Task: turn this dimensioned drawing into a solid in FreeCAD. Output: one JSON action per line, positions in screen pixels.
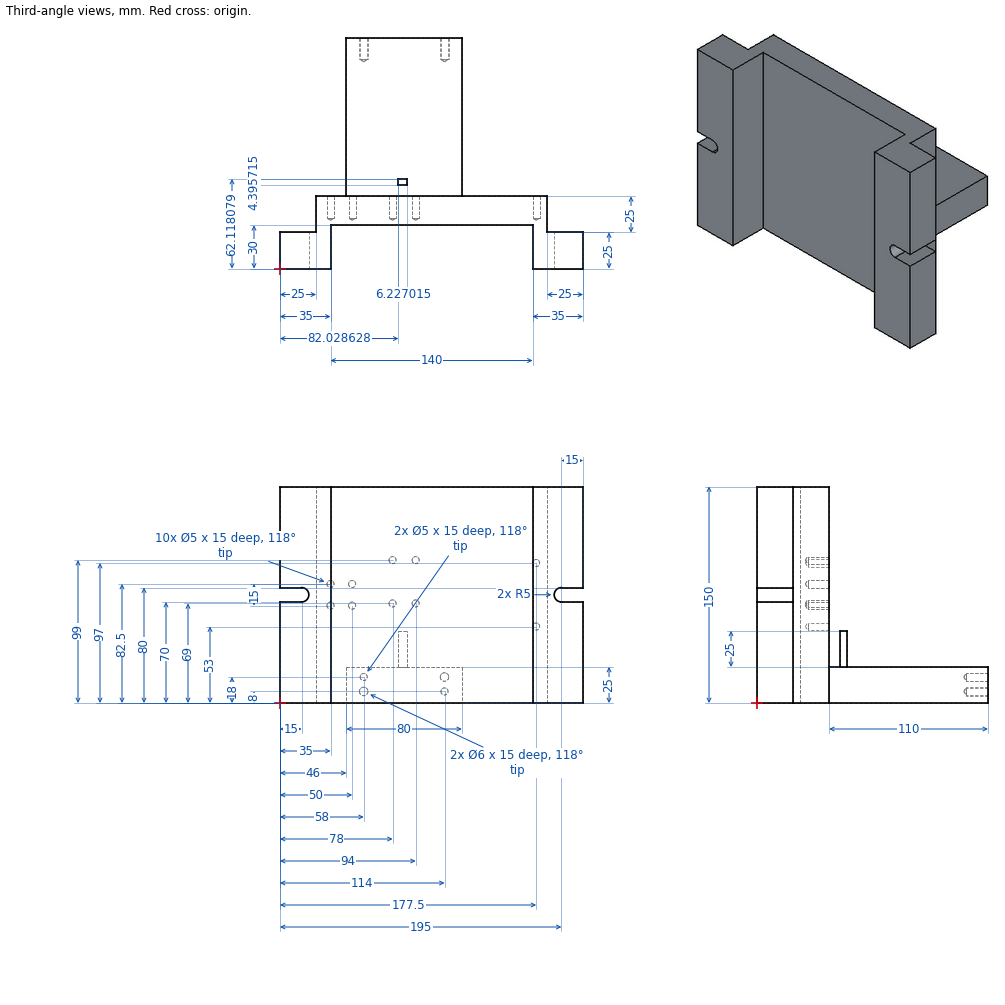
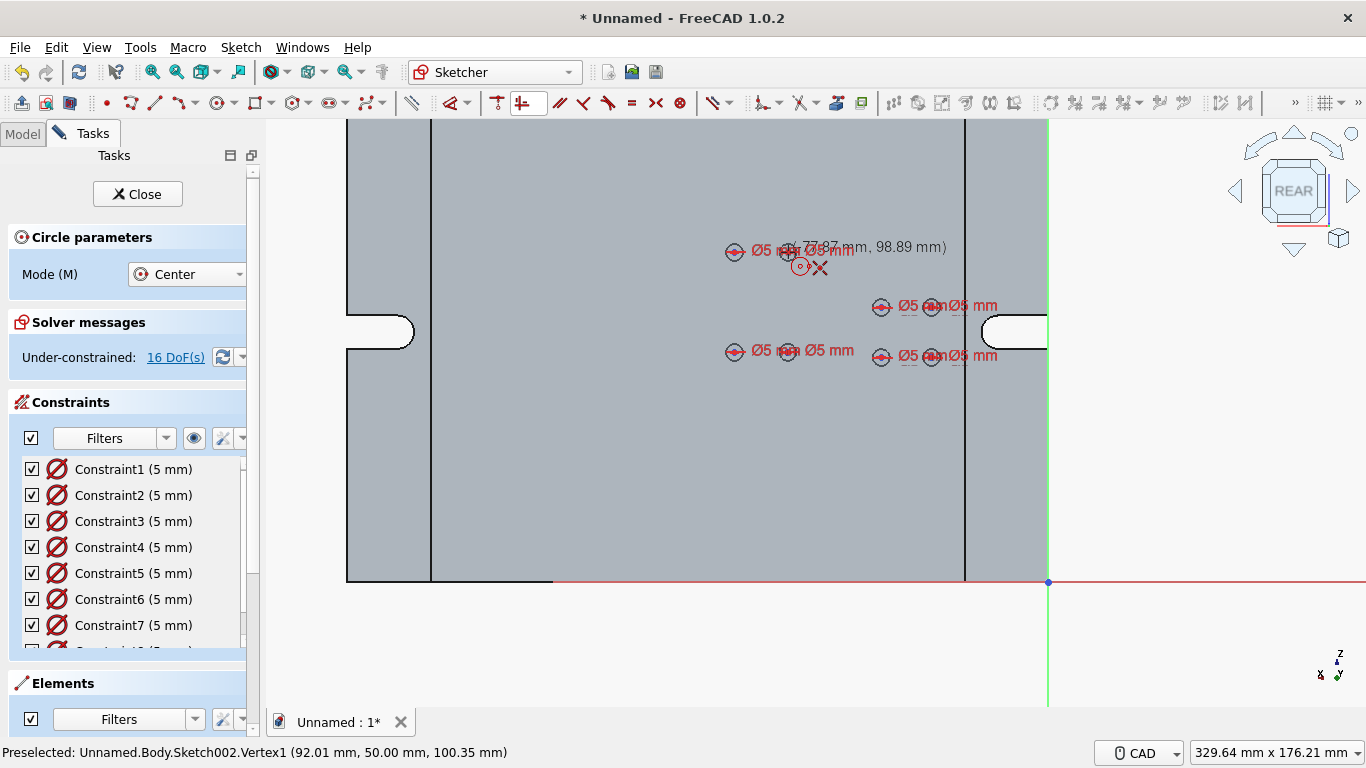
{"action": "scroll", "coordinate": [456, 259], "scroll_direction": "up", "scroll_amount": 6}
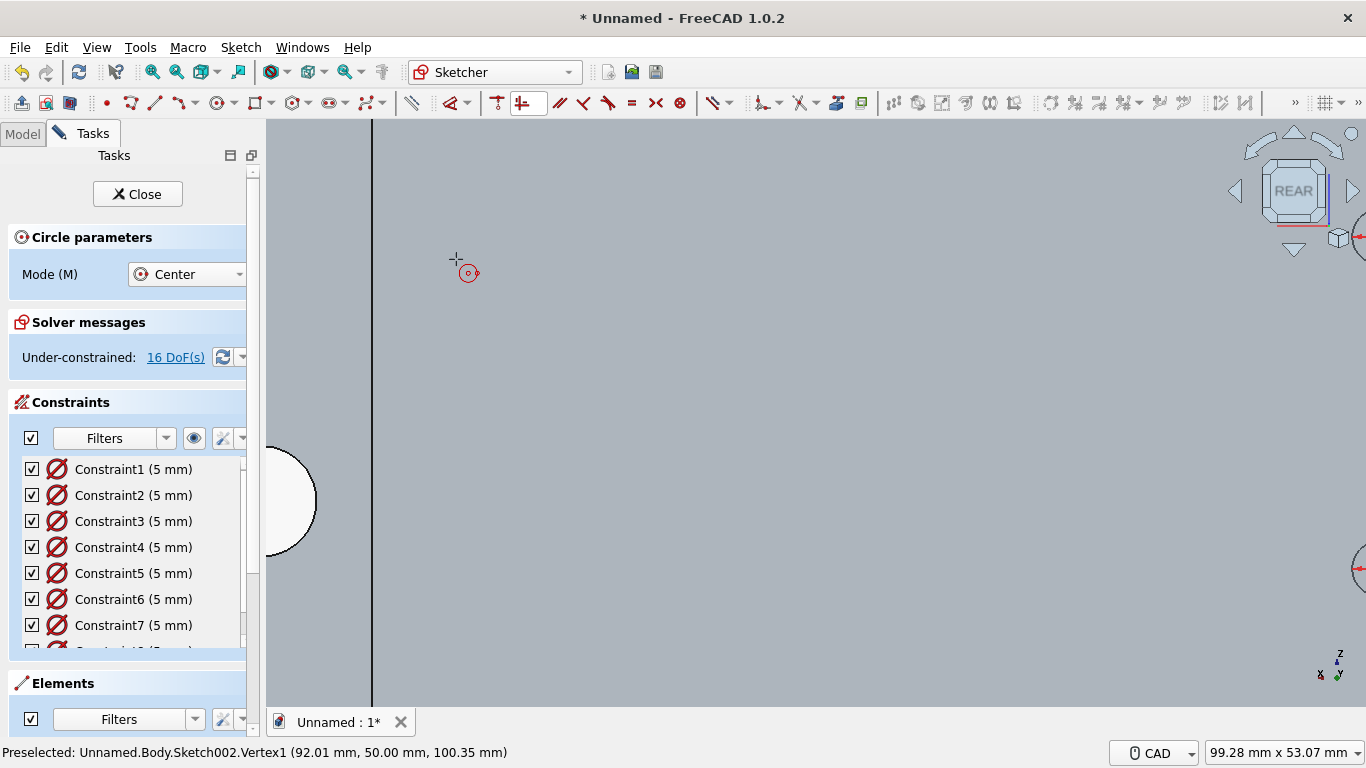
{"action": "left_click", "coordinate": [455, 258]}
{"action": "mouse_move", "coordinate": [475, 238]}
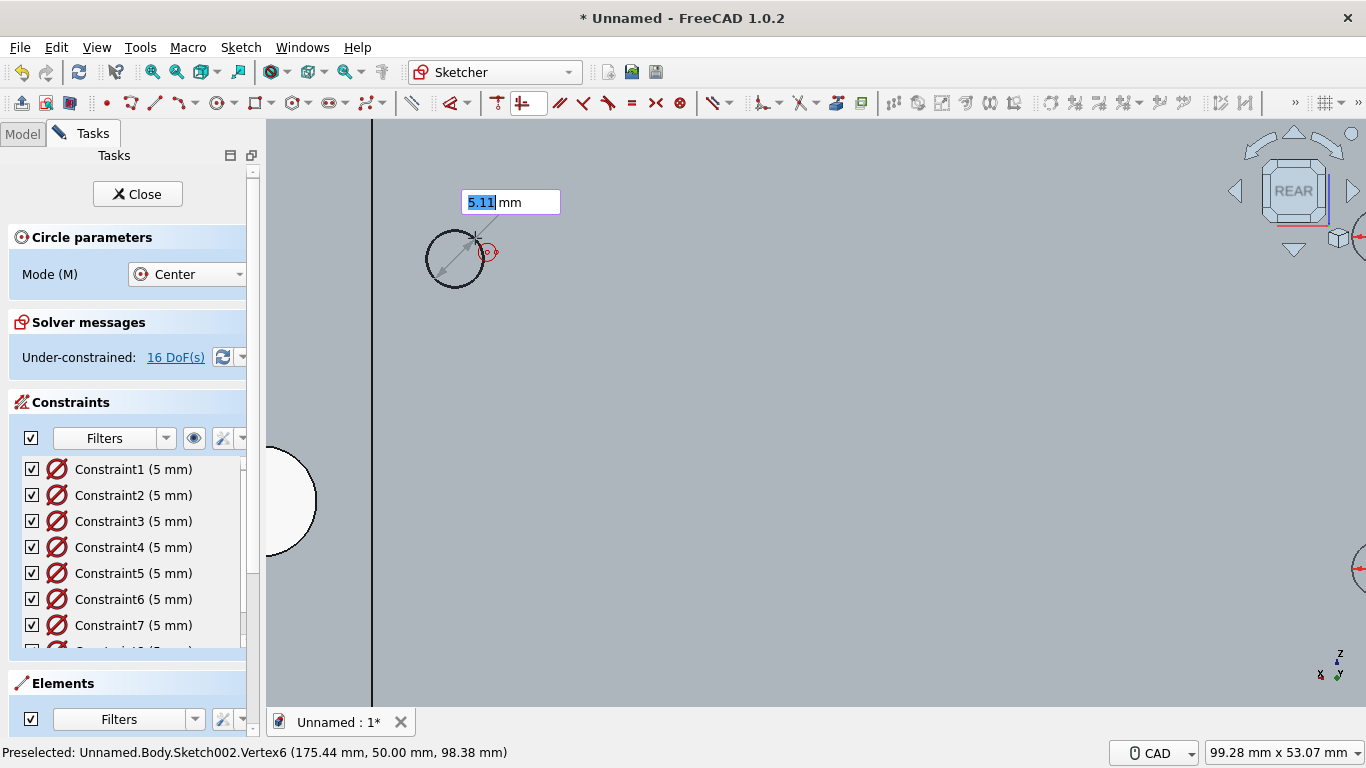
{"action": "type", "text": "5"}
{"action": "key", "text": "Return"}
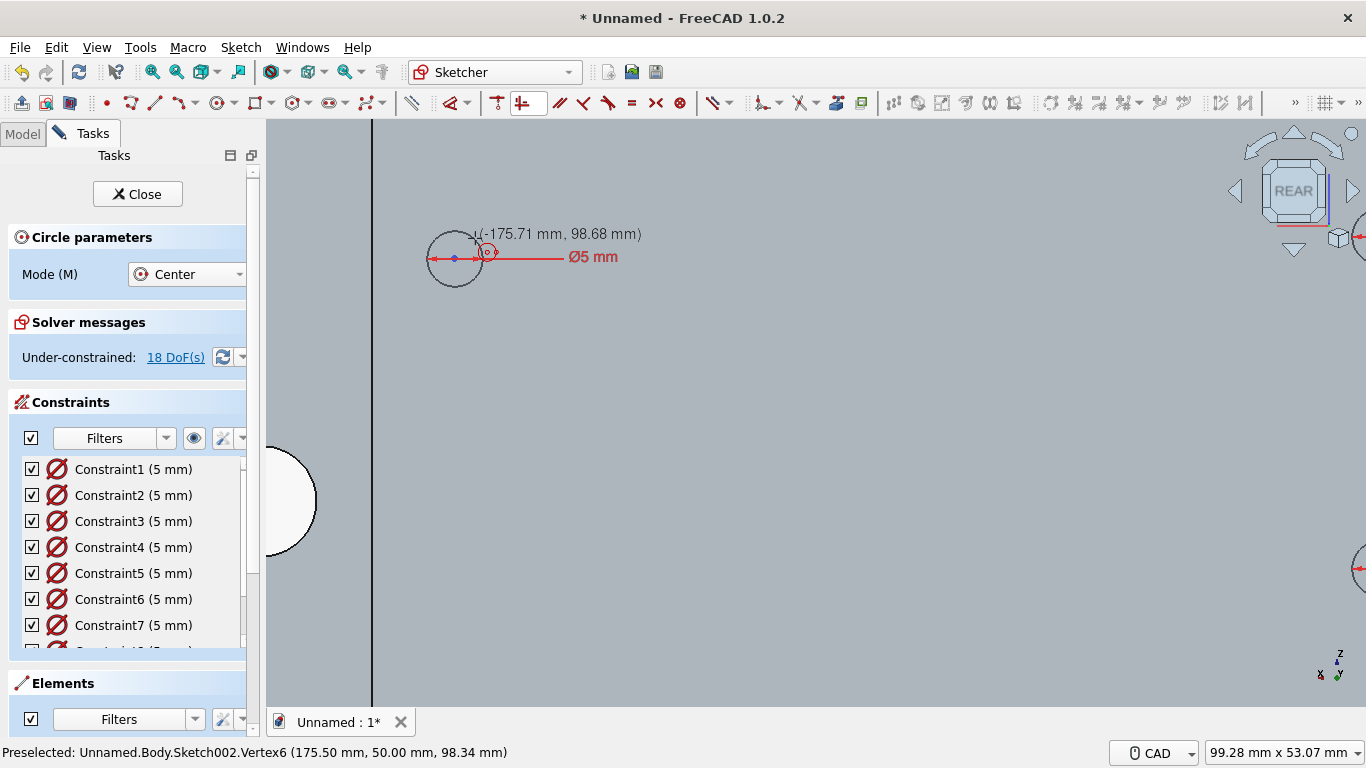
{"action": "scroll", "coordinate": [456, 259], "scroll_direction": "down", "scroll_amount": 6}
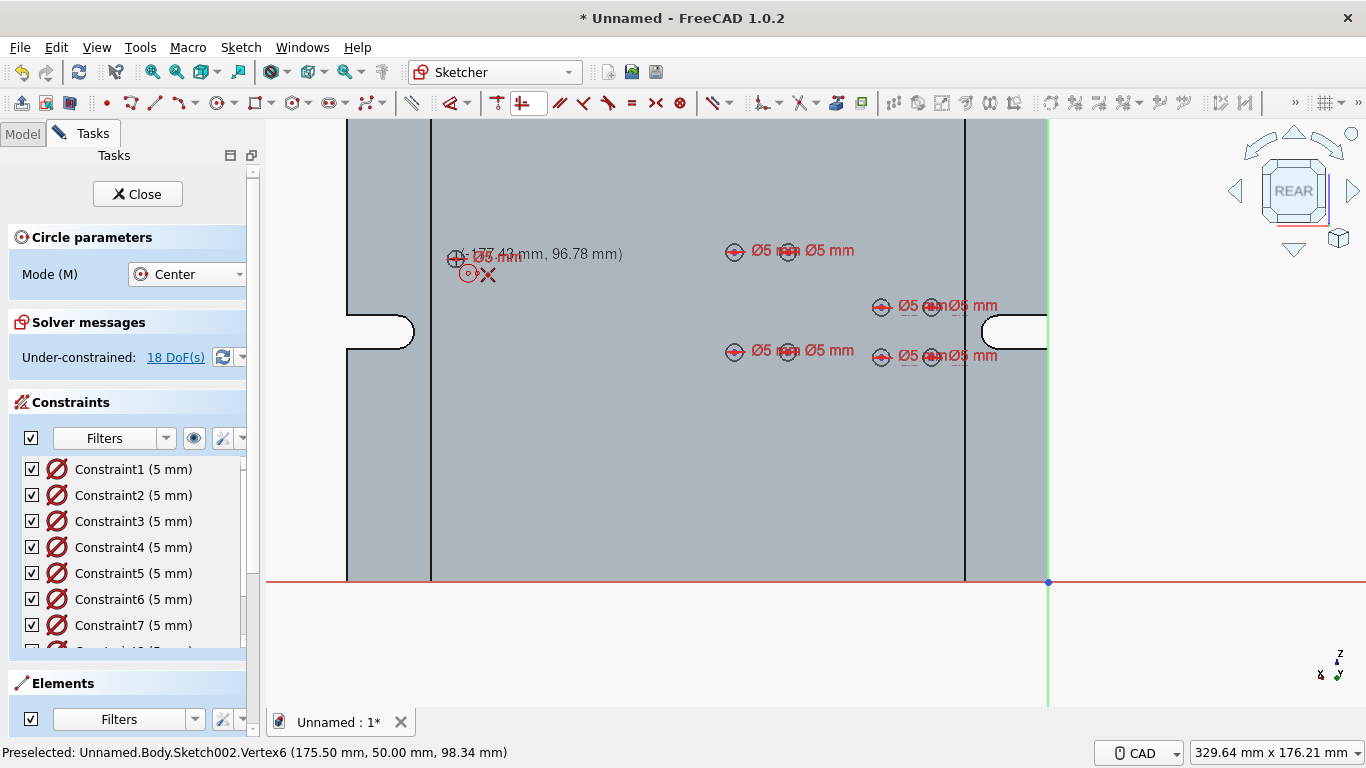
{"action": "scroll", "coordinate": [456, 406], "scroll_direction": "up", "scroll_amount": 6}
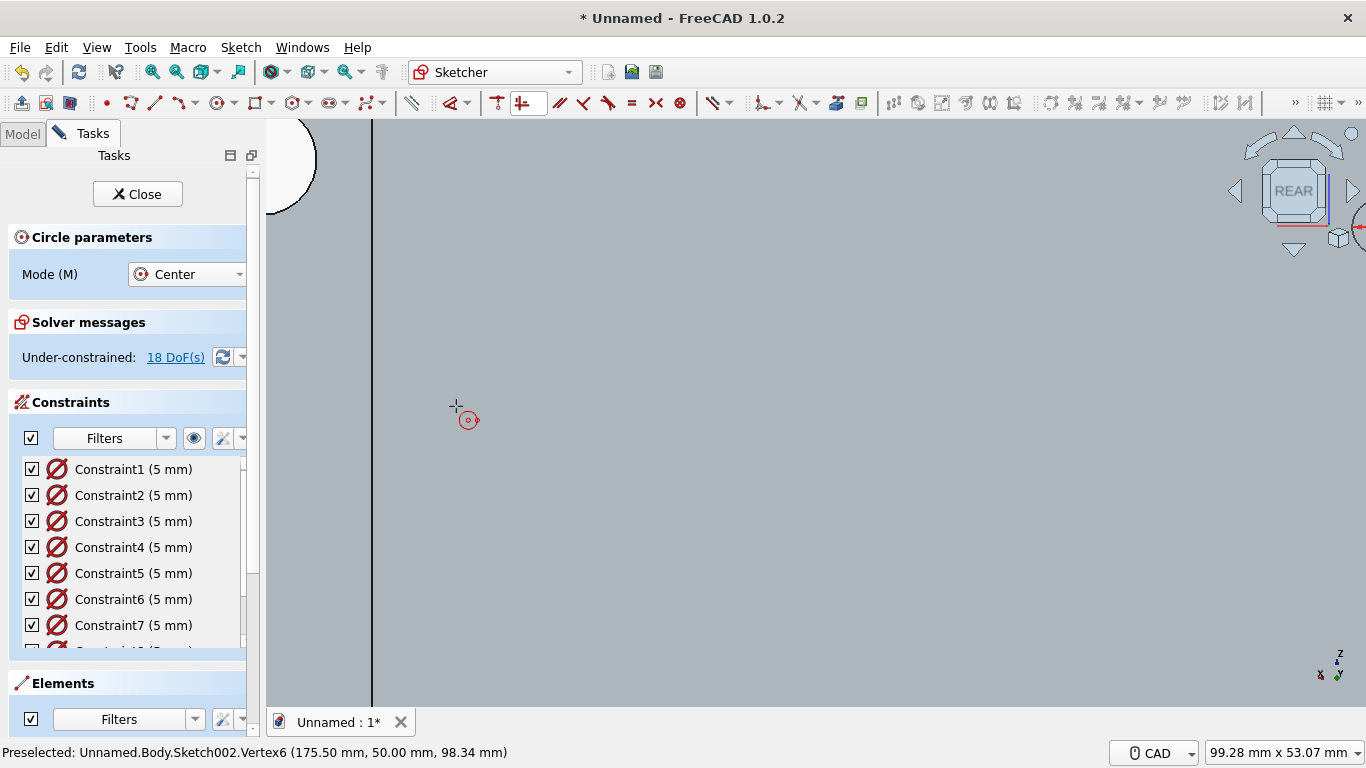
{"action": "left_click", "coordinate": [455, 403]}
{"action": "mouse_move", "coordinate": [475, 384]}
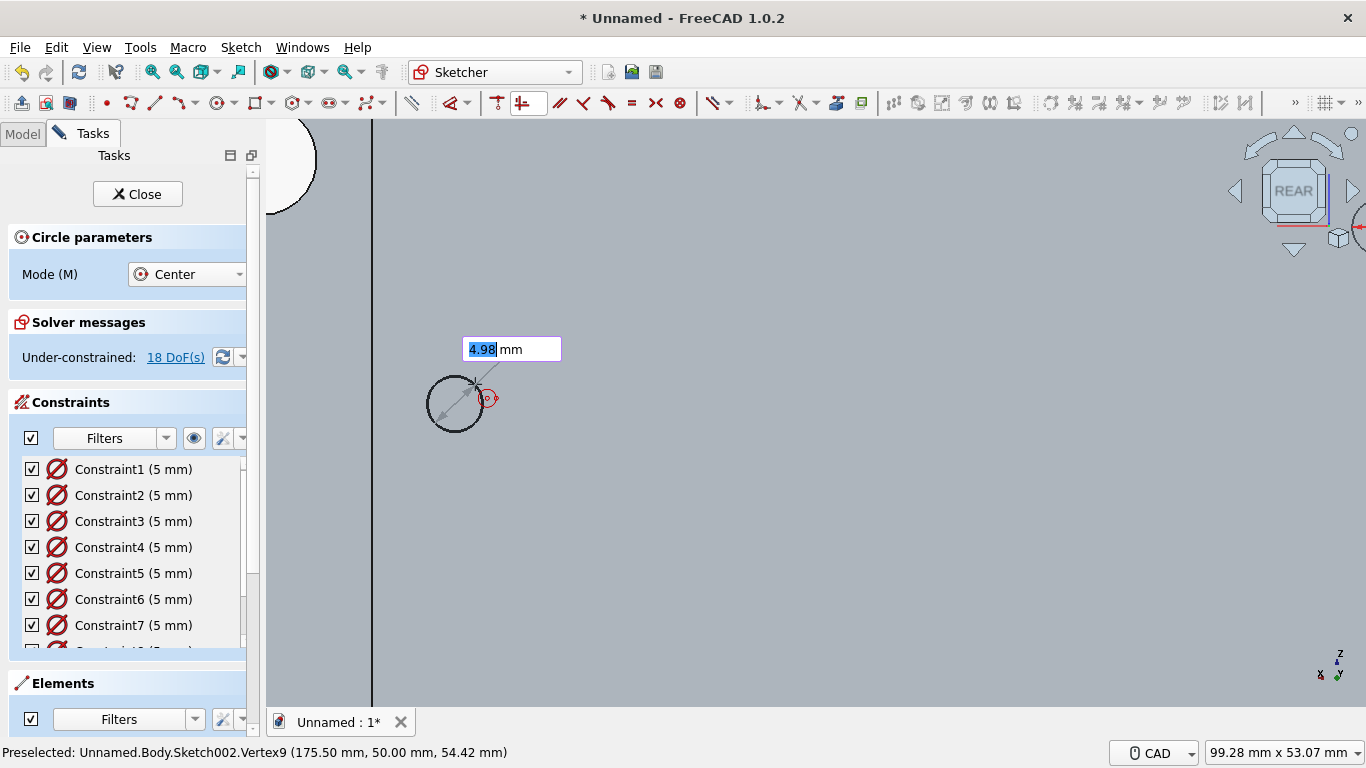
{"action": "type", "text": "5"}
{"action": "key", "text": "Return"}
{"action": "key", "text": "Escape"}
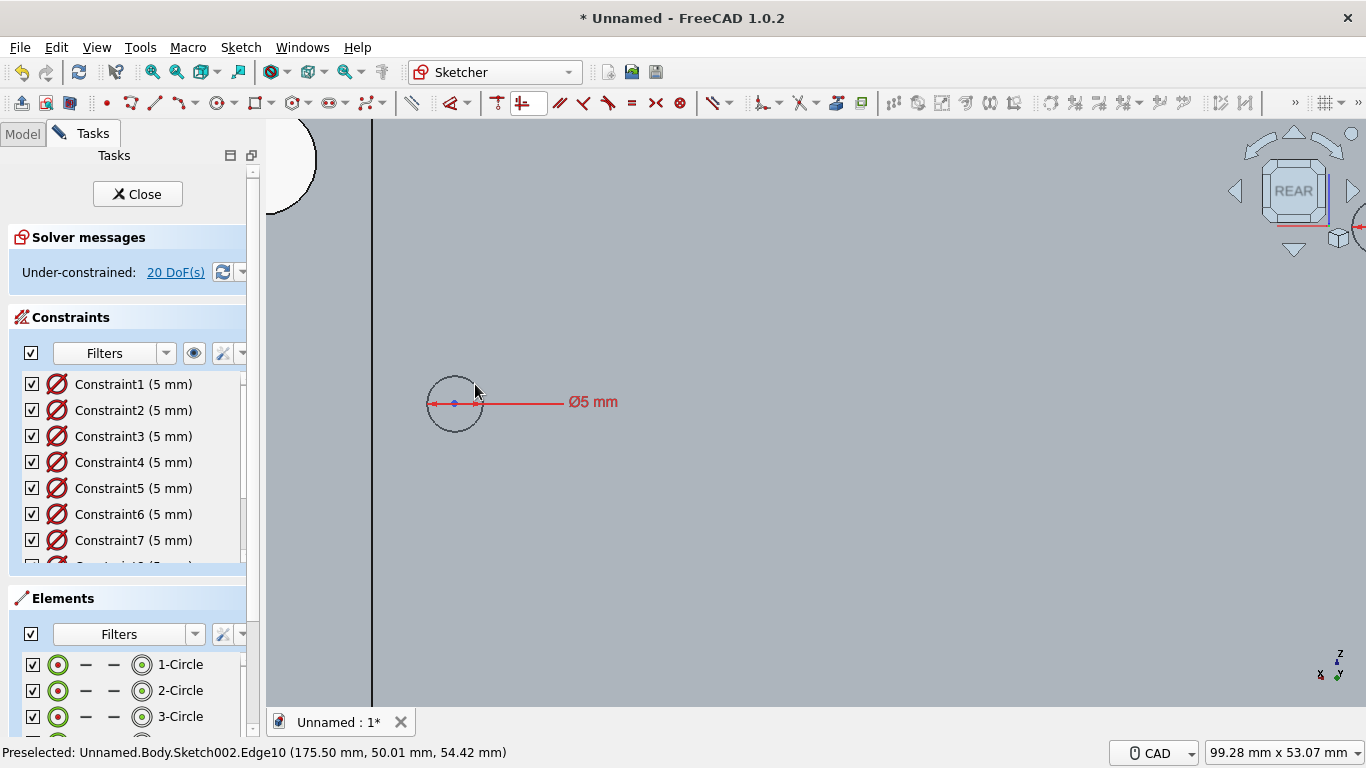
{"action": "scroll", "coordinate": [456, 406], "scroll_direction": "down", "scroll_amount": 6}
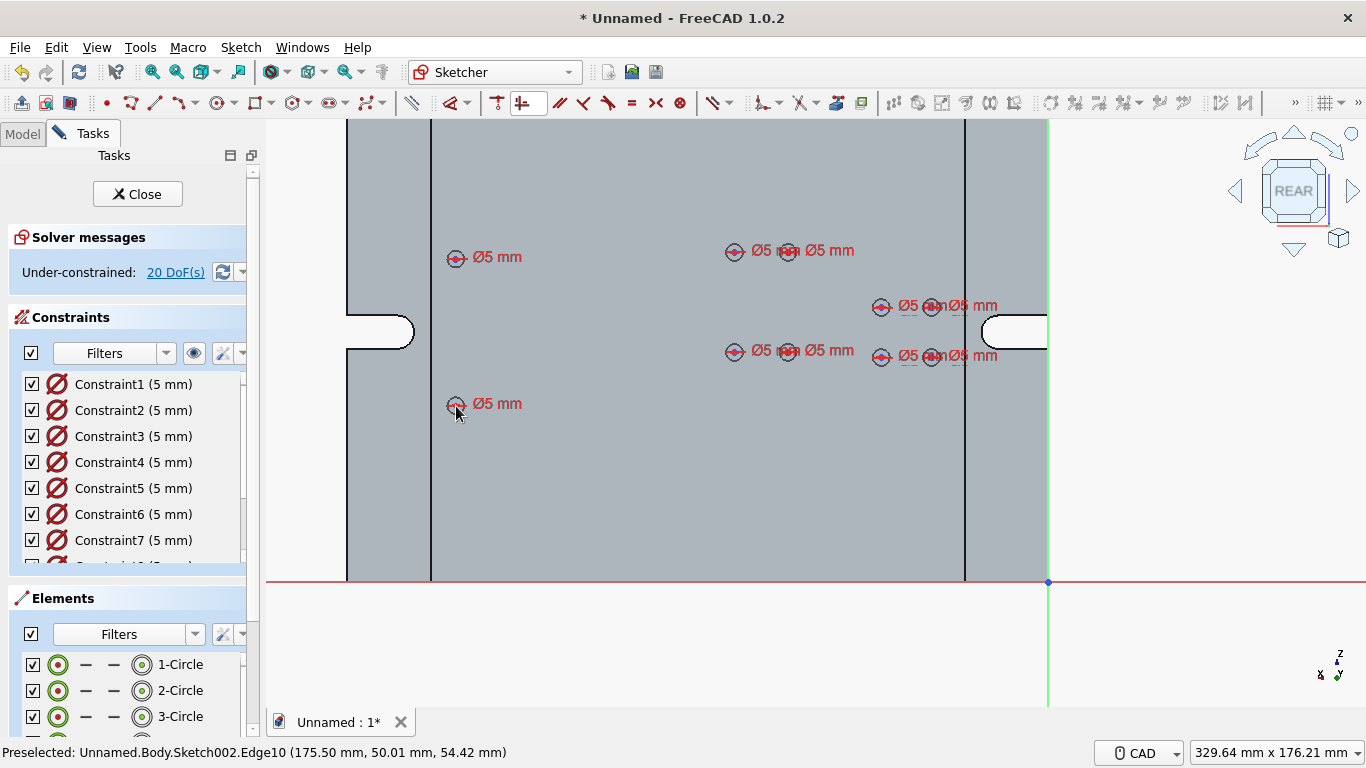
{"action": "left_click", "coordinate": [932, 308]}